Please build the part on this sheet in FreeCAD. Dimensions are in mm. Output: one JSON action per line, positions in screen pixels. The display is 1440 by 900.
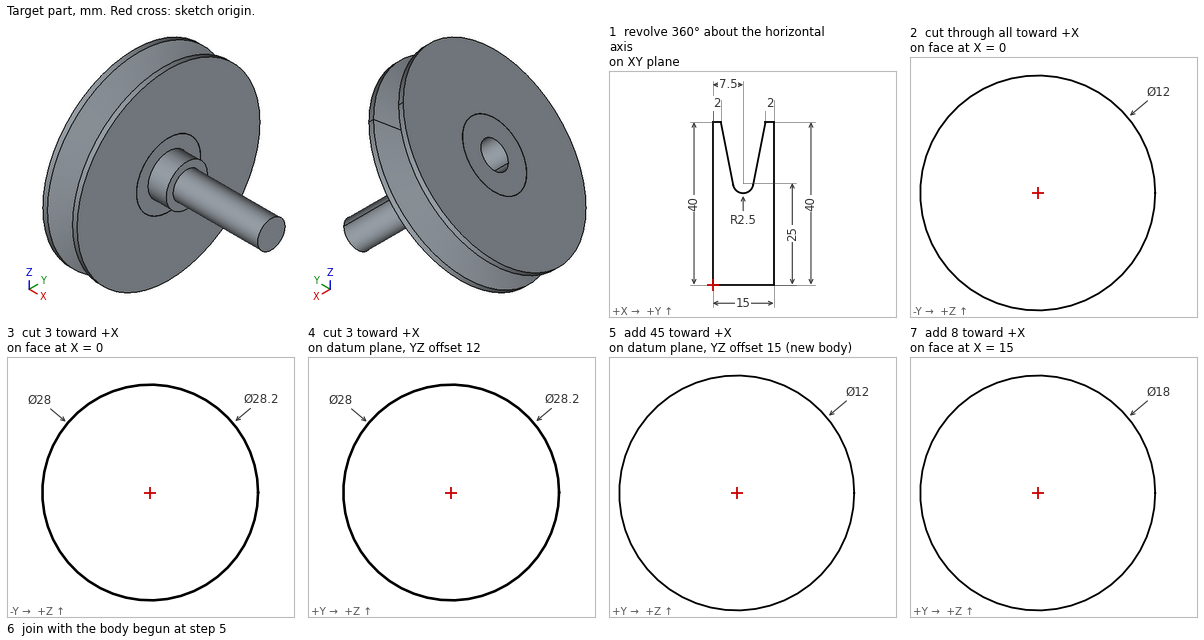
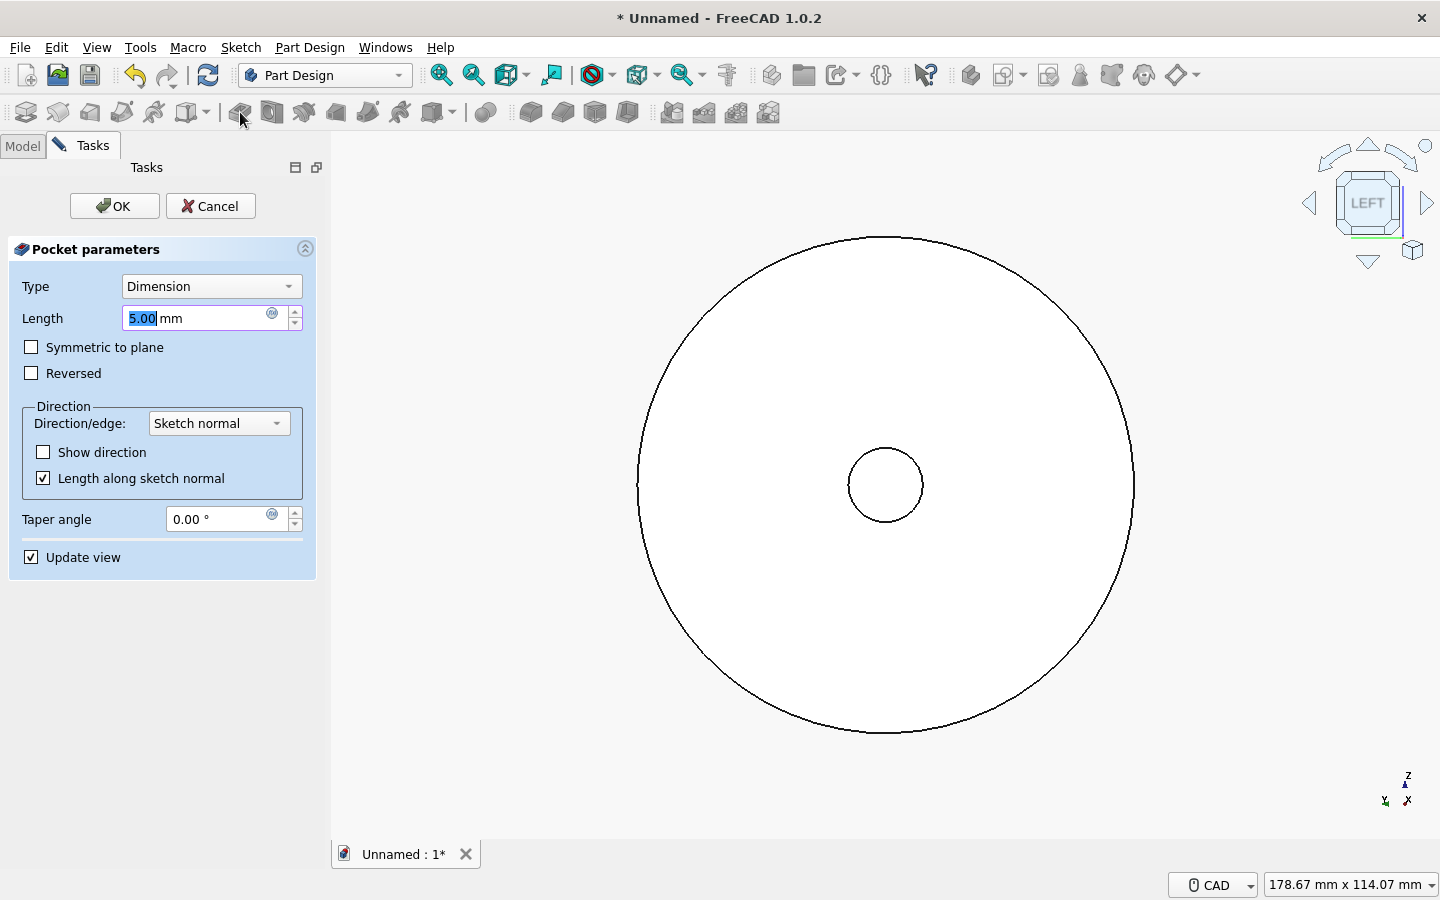
{"action": "left_click", "coordinate": [212, 286]}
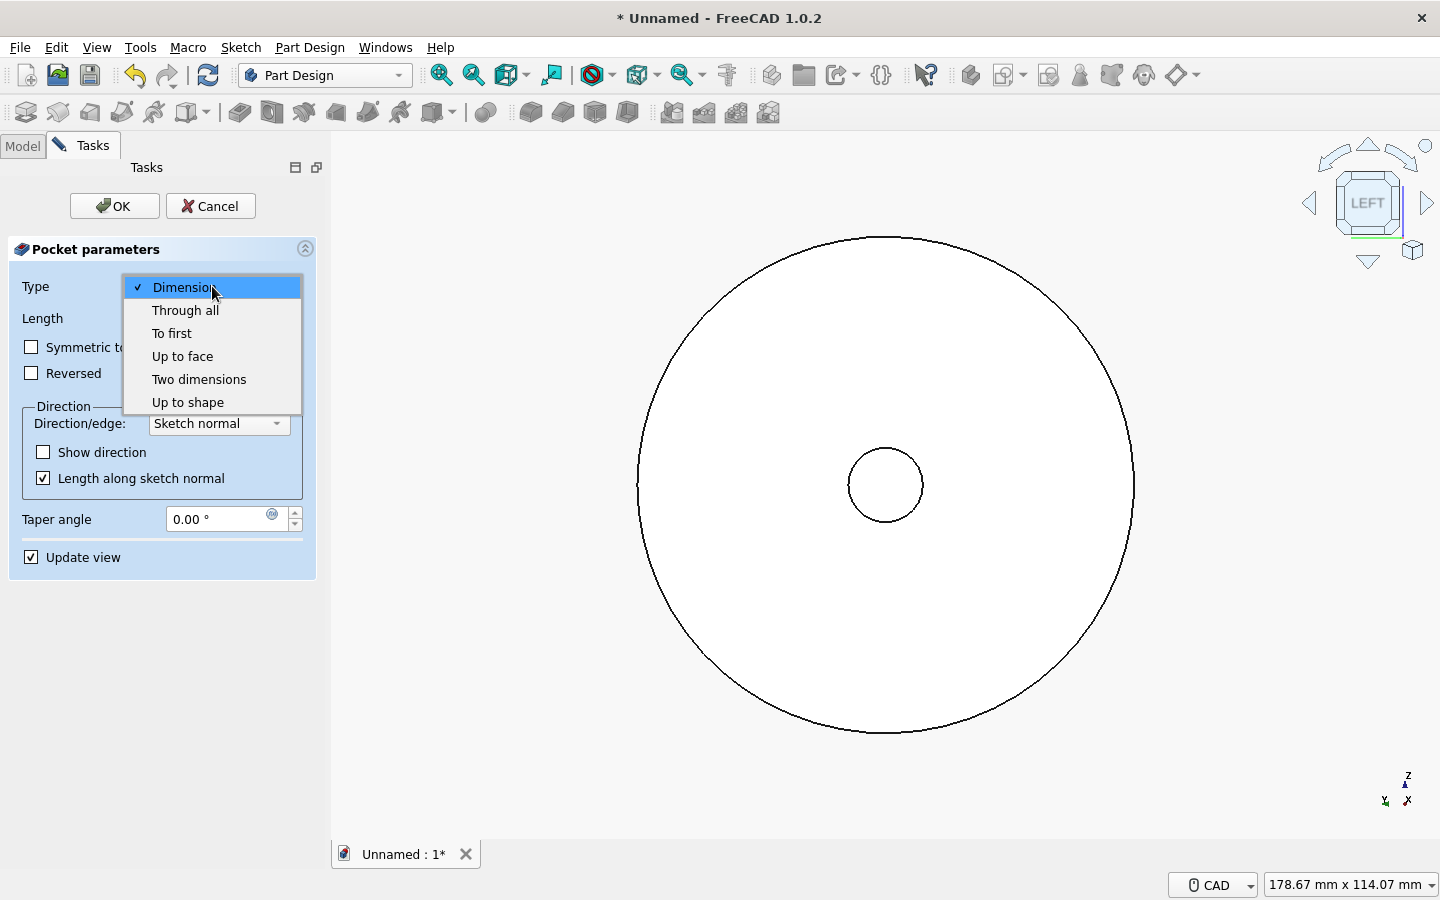
{"action": "left_click", "coordinate": [212, 310]}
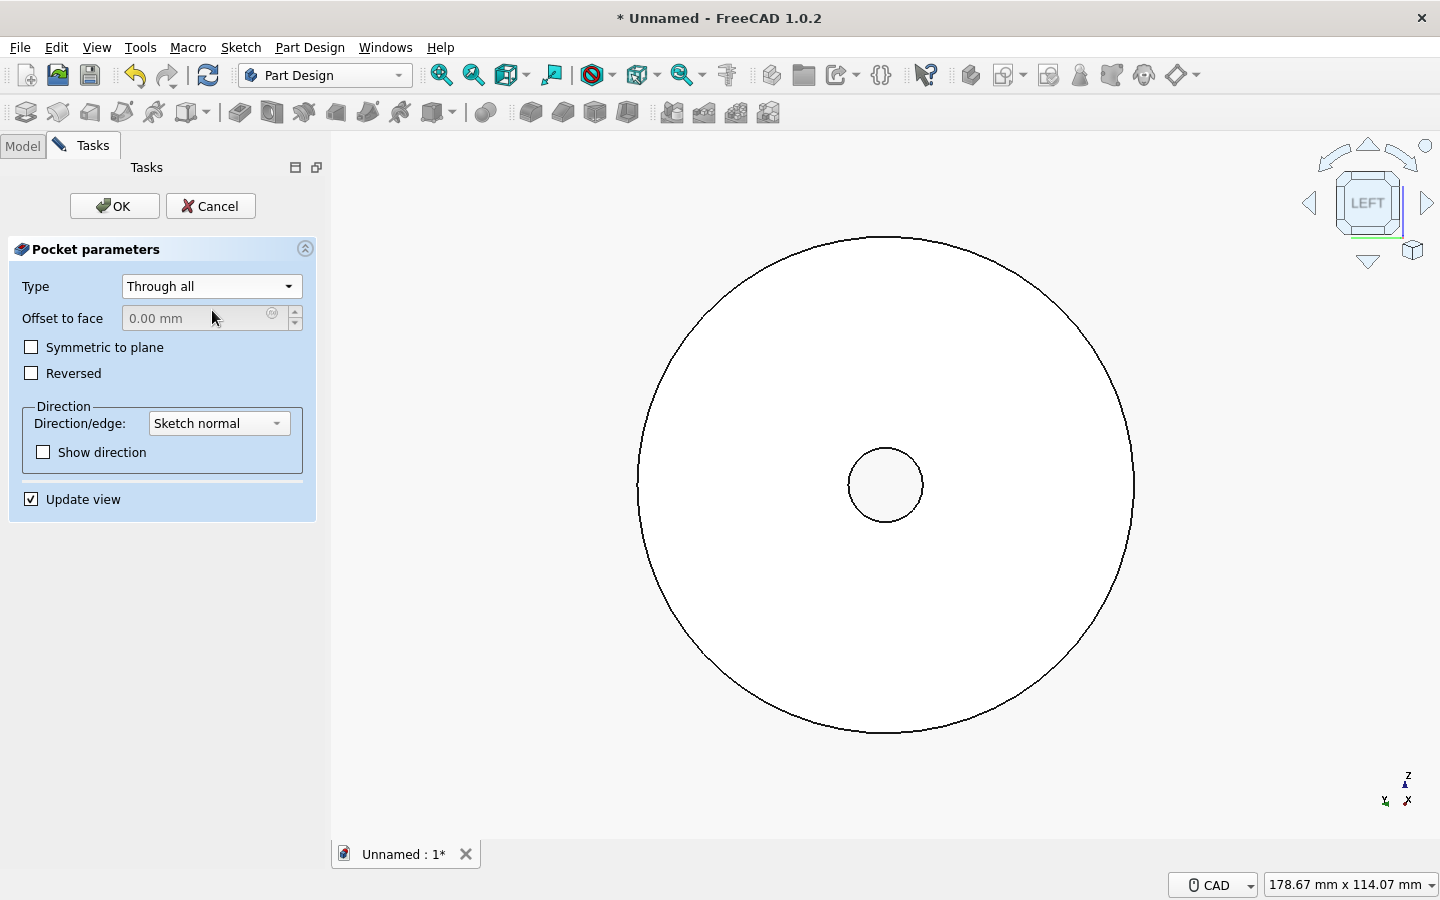
{"action": "left_click", "coordinate": [115, 206]}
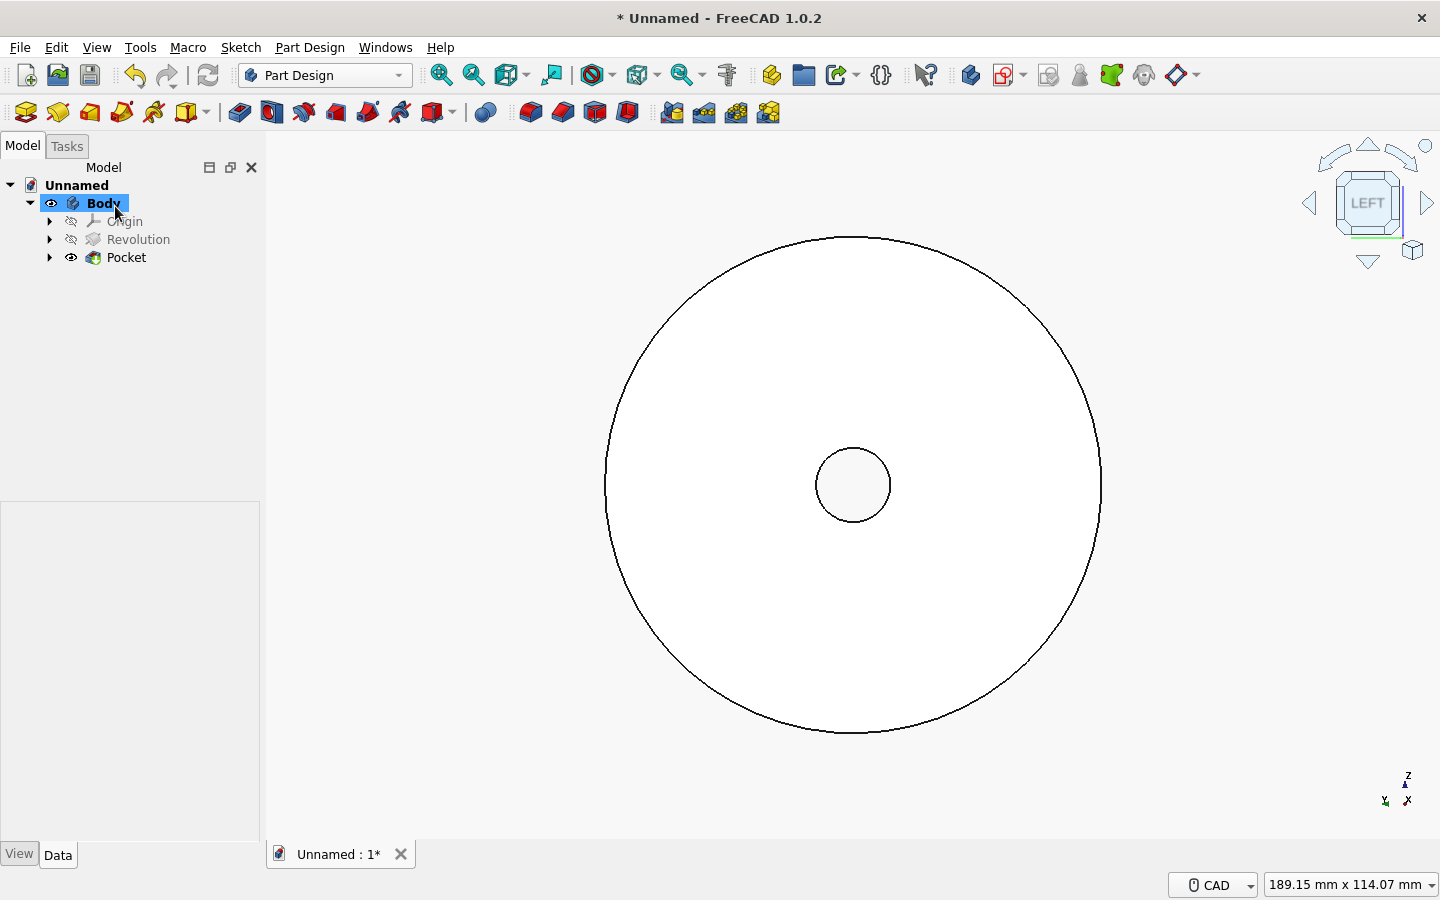
{"action": "left_click", "coordinate": [853, 626]}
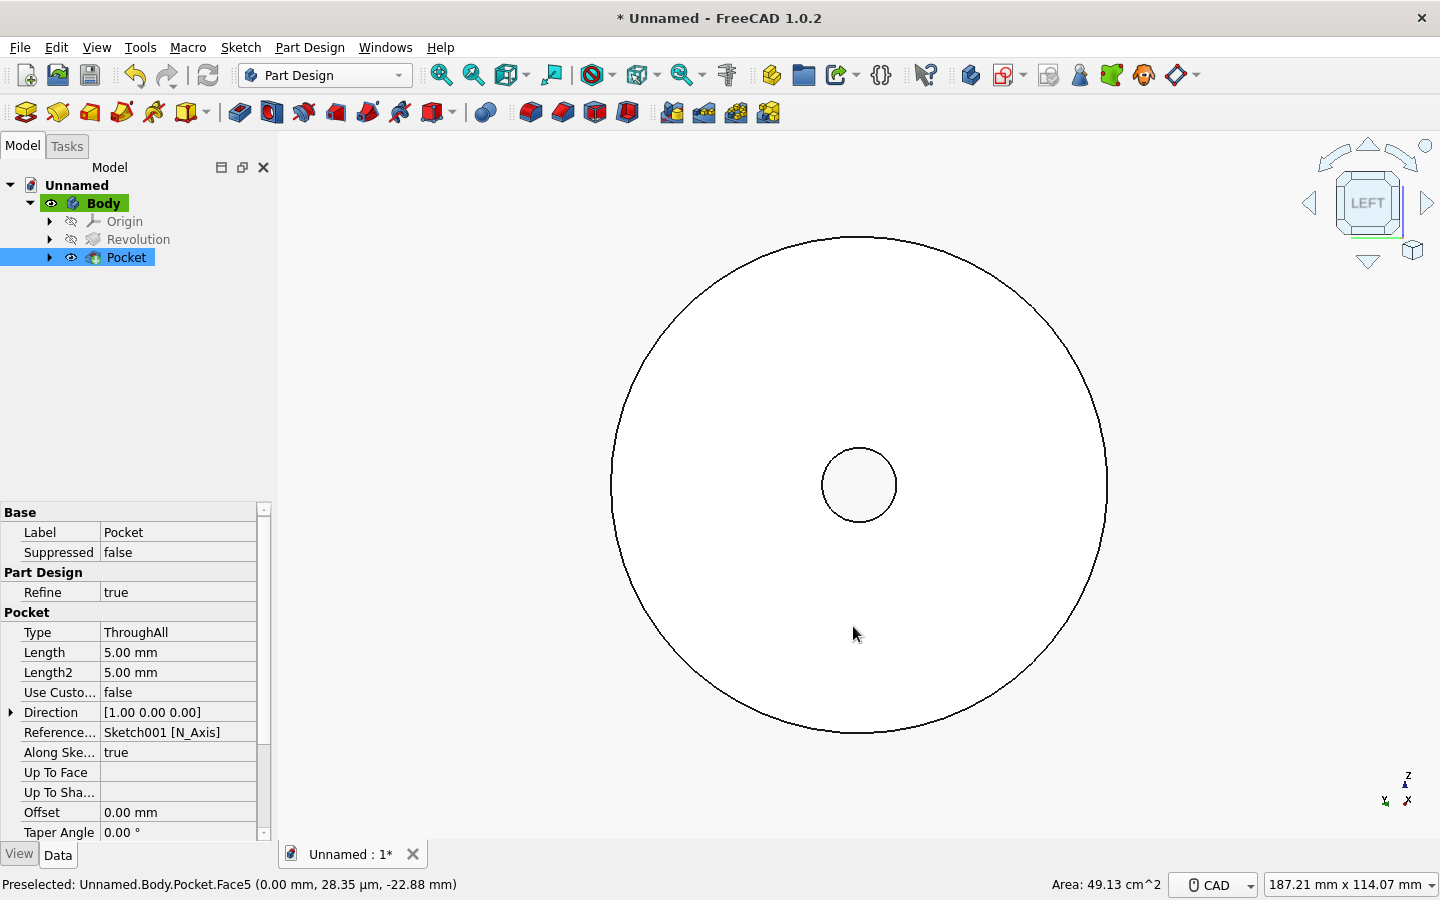
{"action": "left_click", "coordinate": [1004, 76]}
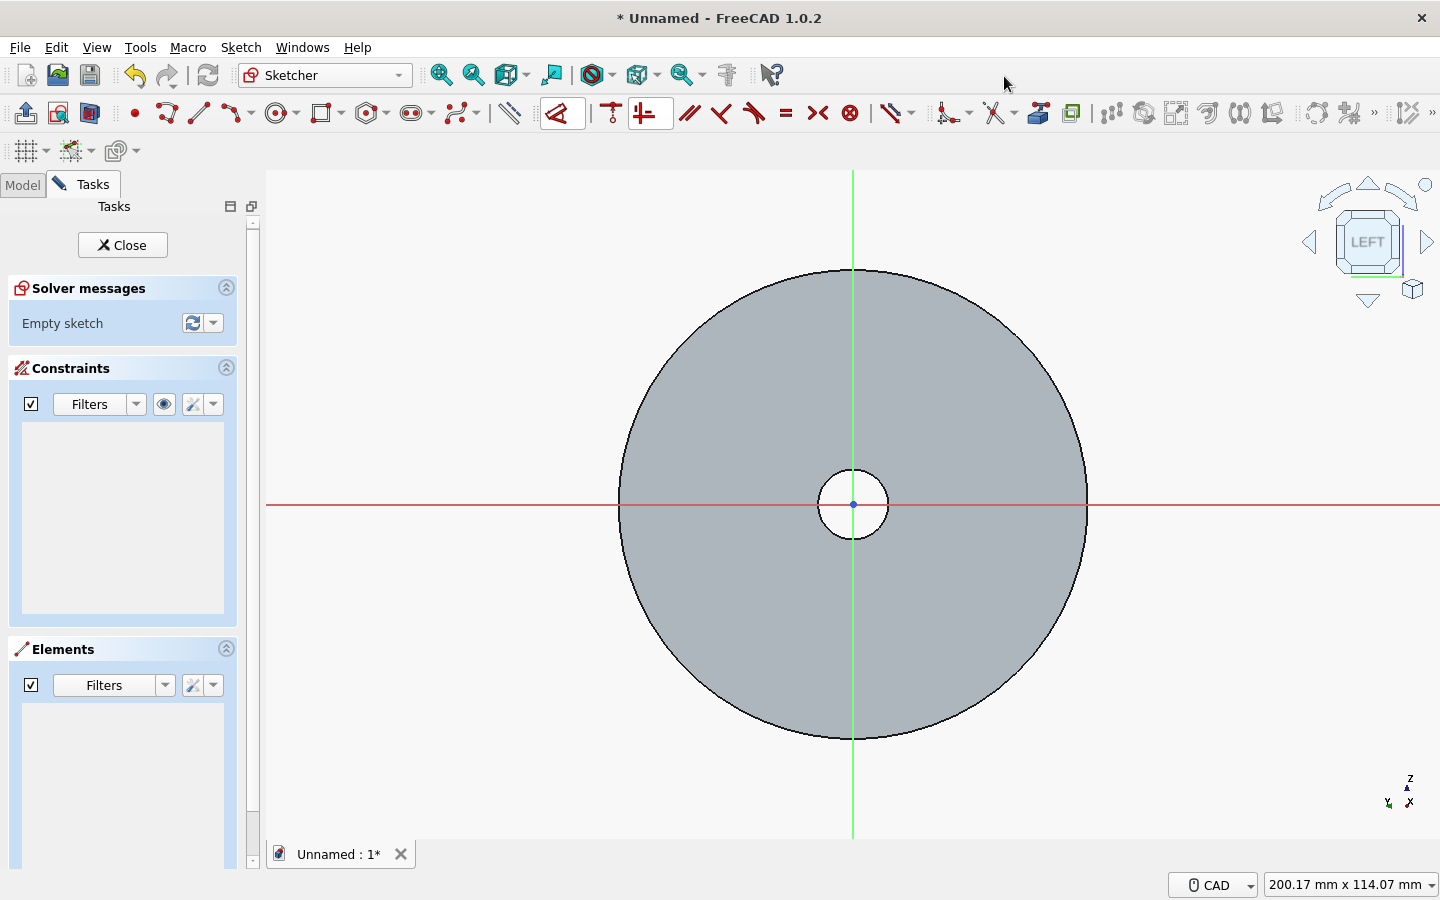
{"action": "scroll", "coordinate": [893, 505], "scroll_direction": "up", "scroll_amount": 5}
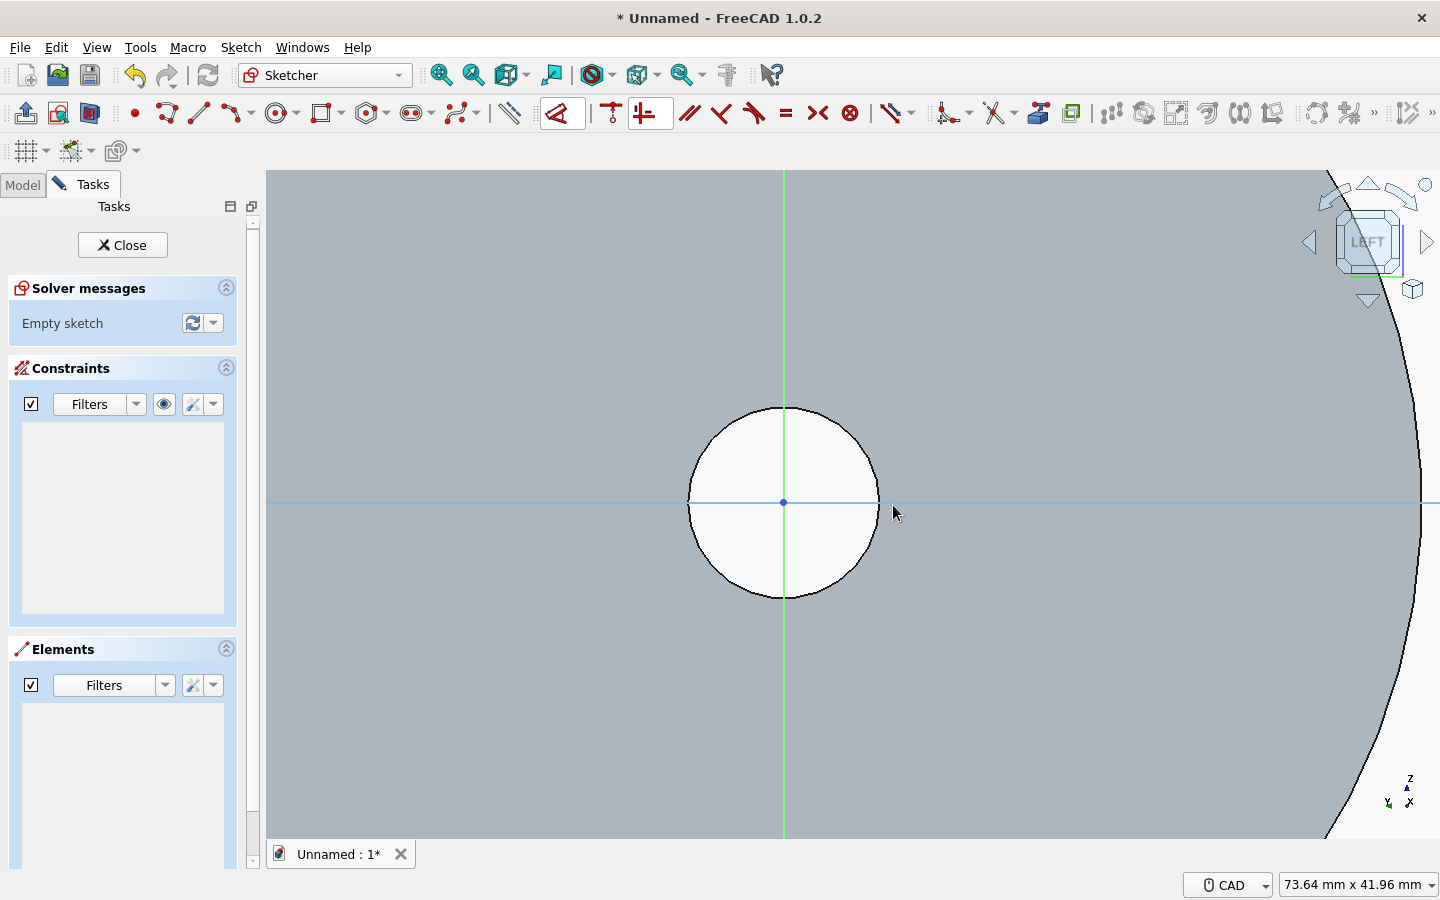
{"action": "left_click", "coordinate": [276, 114]}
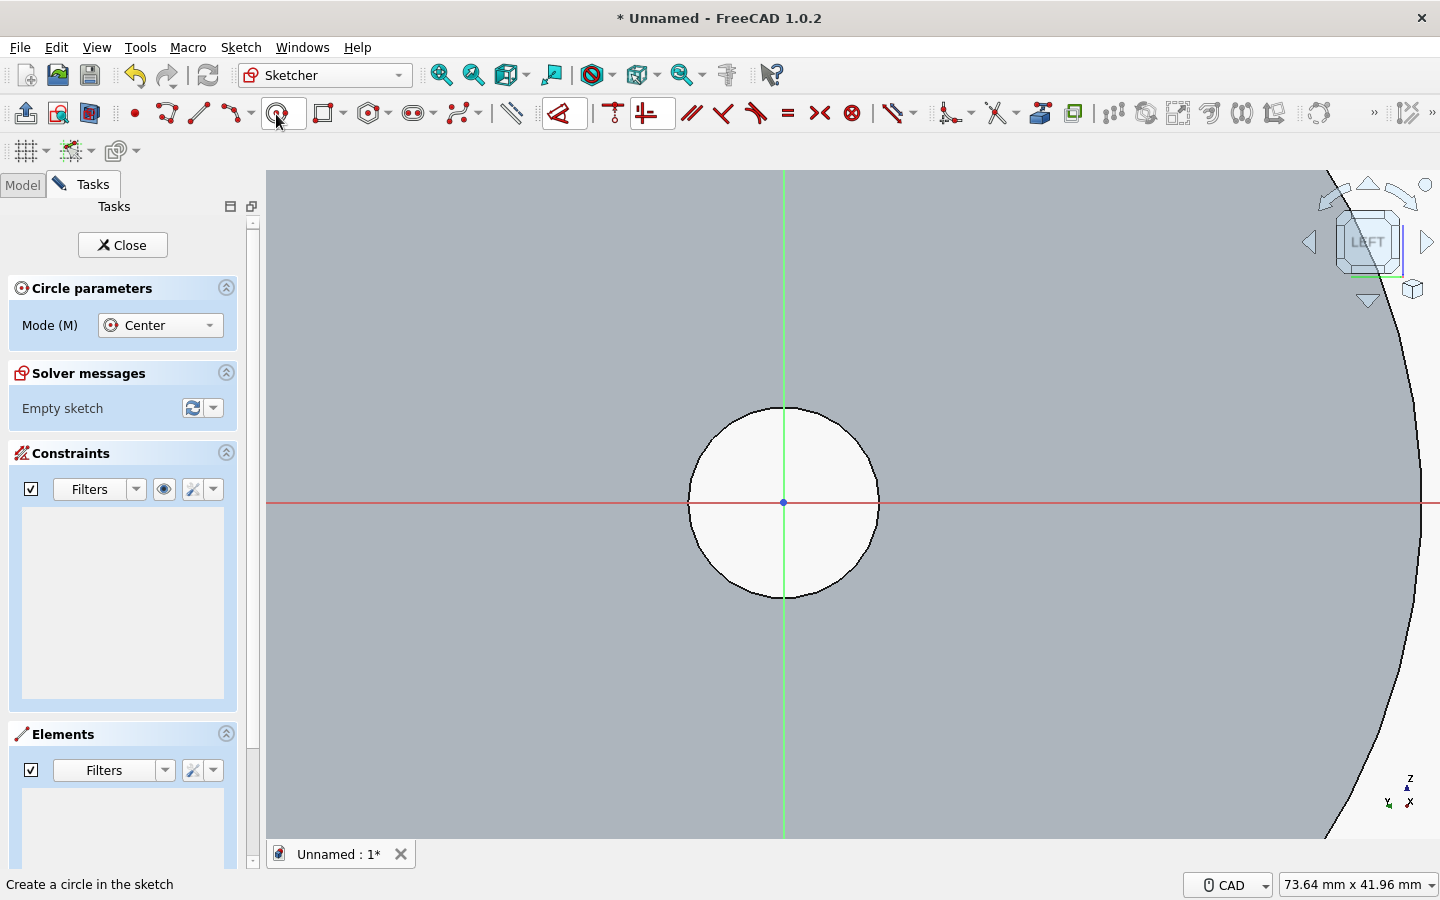
{"action": "left_click", "coordinate": [784, 503]}
{"action": "mouse_move", "coordinate": [943, 344]}